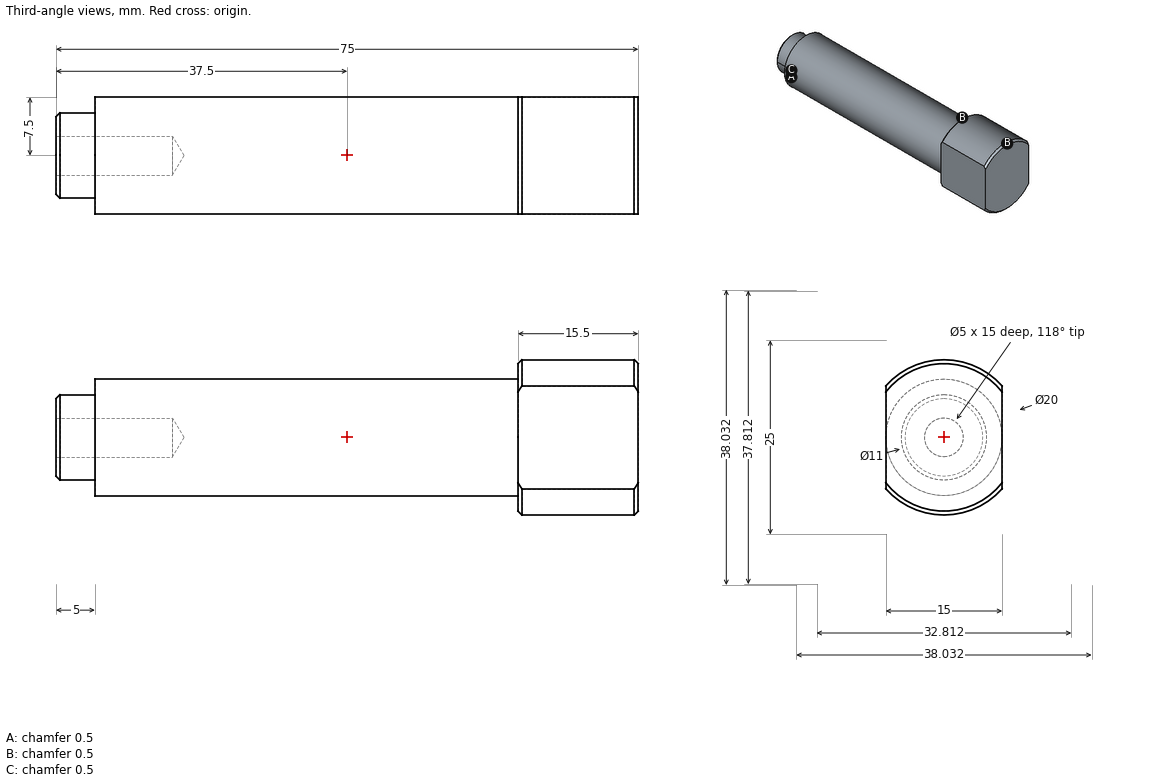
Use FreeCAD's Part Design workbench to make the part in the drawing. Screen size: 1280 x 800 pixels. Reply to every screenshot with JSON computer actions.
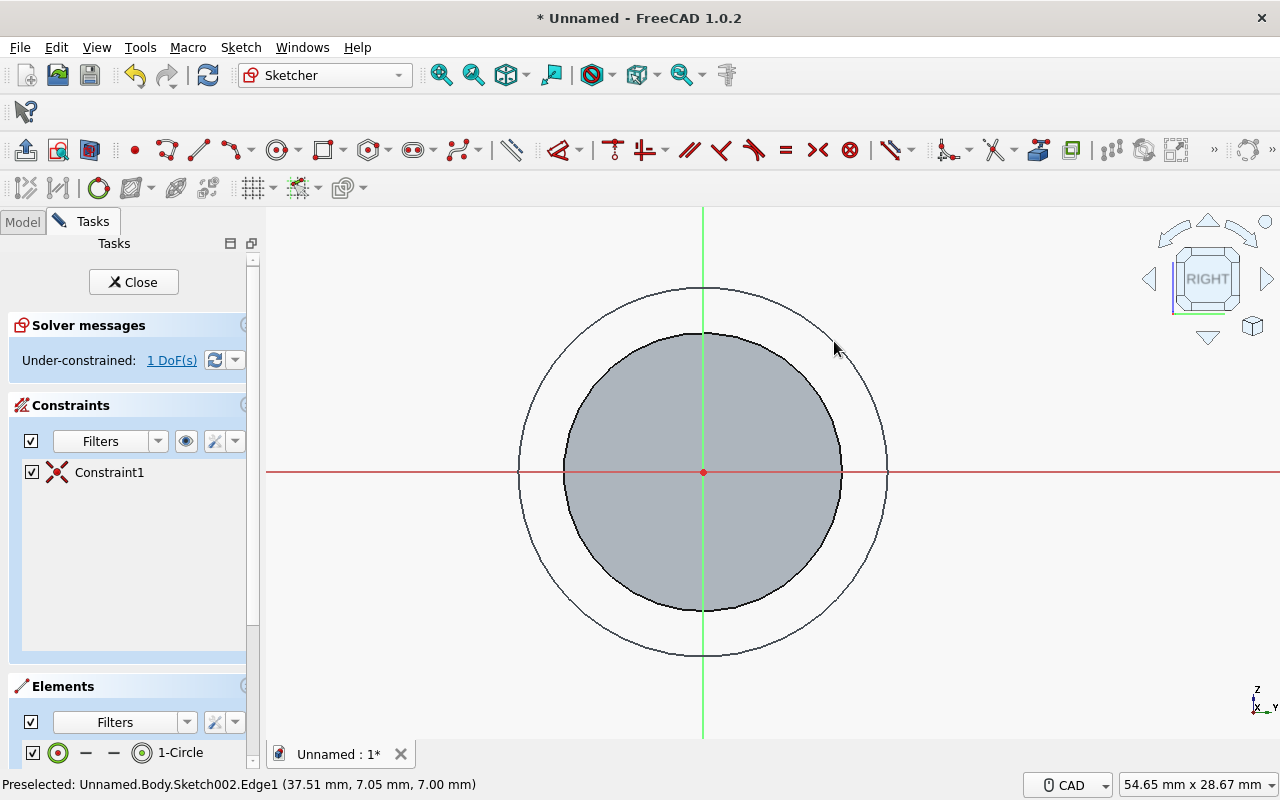
{"action": "left_click", "coordinate": [558, 150]}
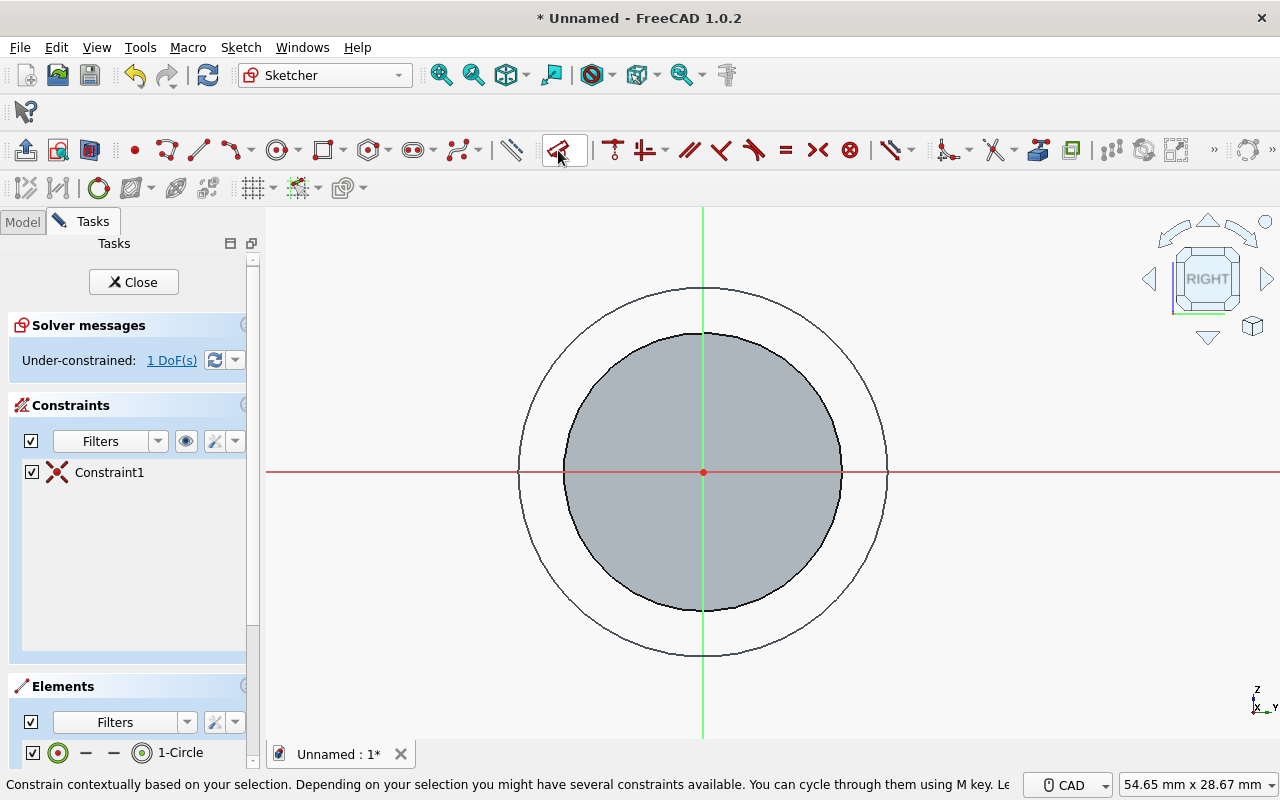
{"action": "left_click", "coordinate": [833, 341]}
{"action": "left_click", "coordinate": [856, 318]}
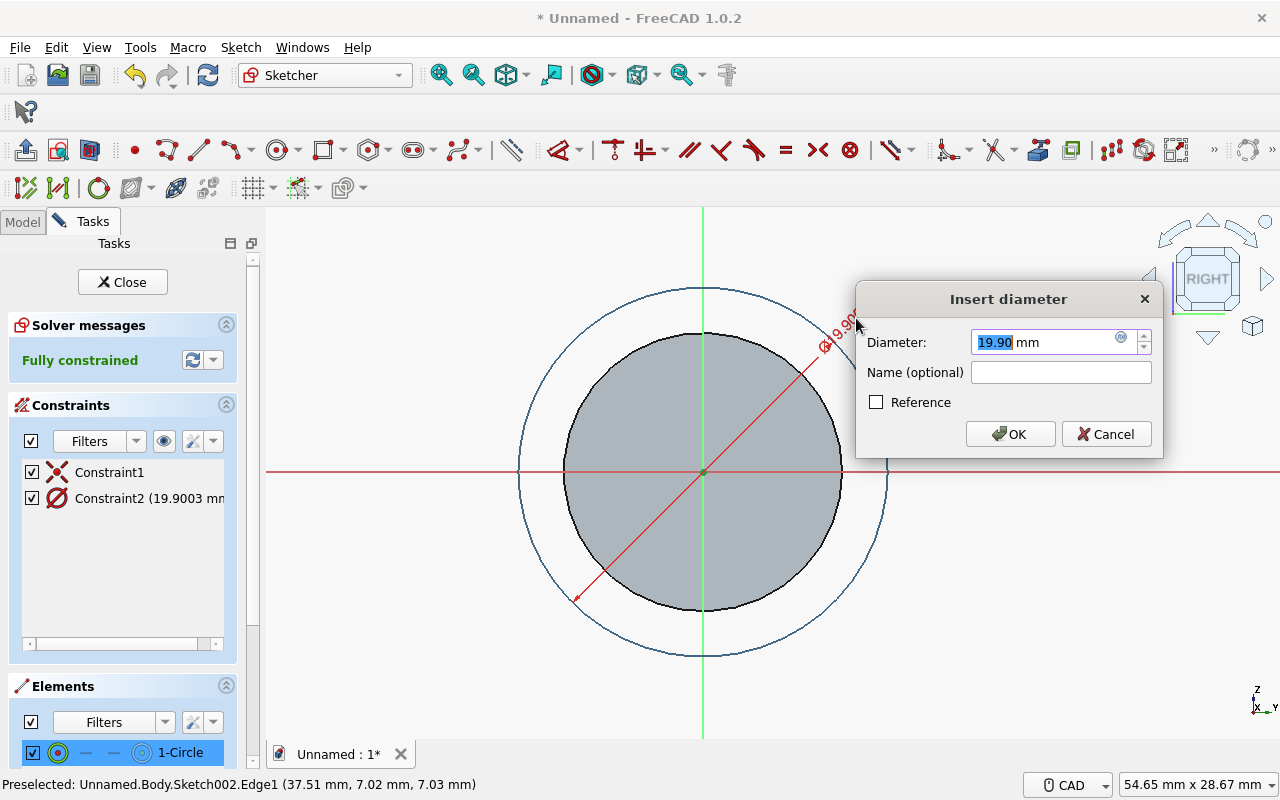
{"action": "type", "text": "20"}
{"action": "key", "text": "Return"}
{"action": "key", "text": "Escape"}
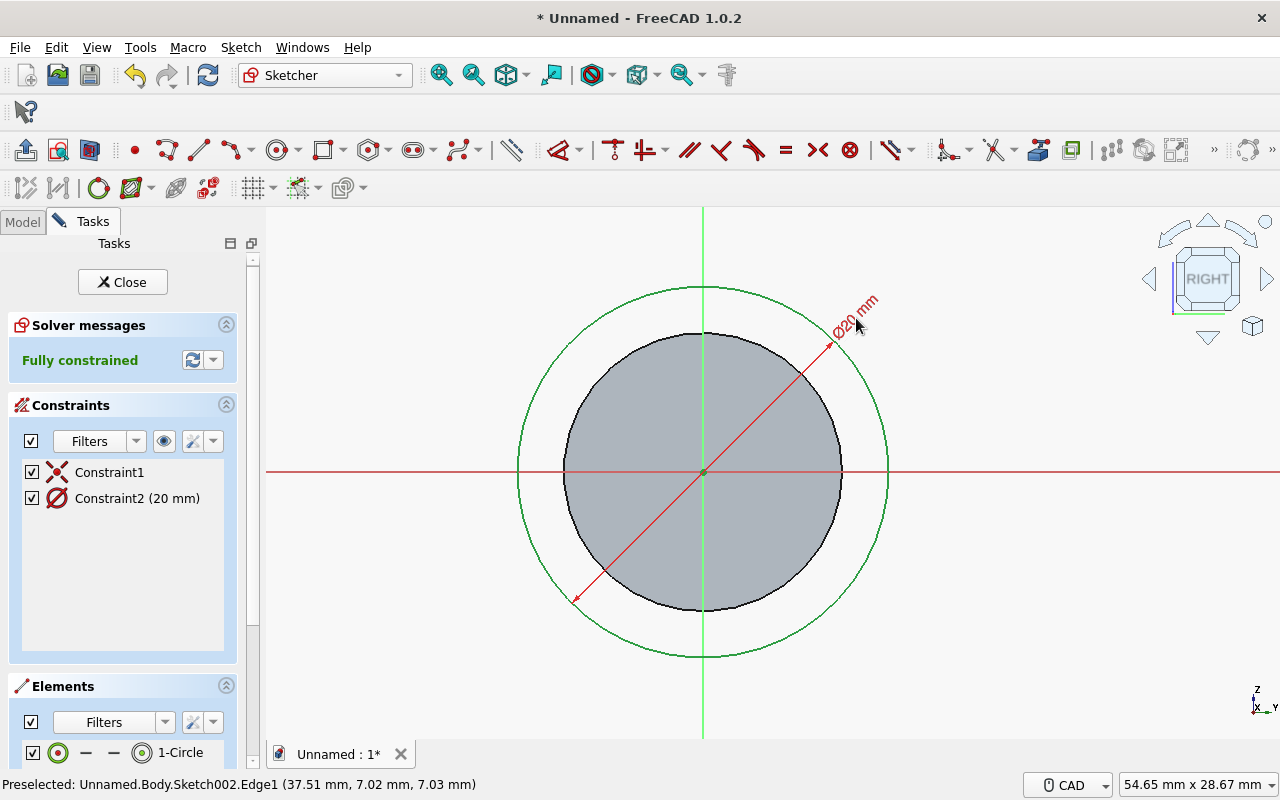
{"action": "left_click", "coordinate": [123, 282]}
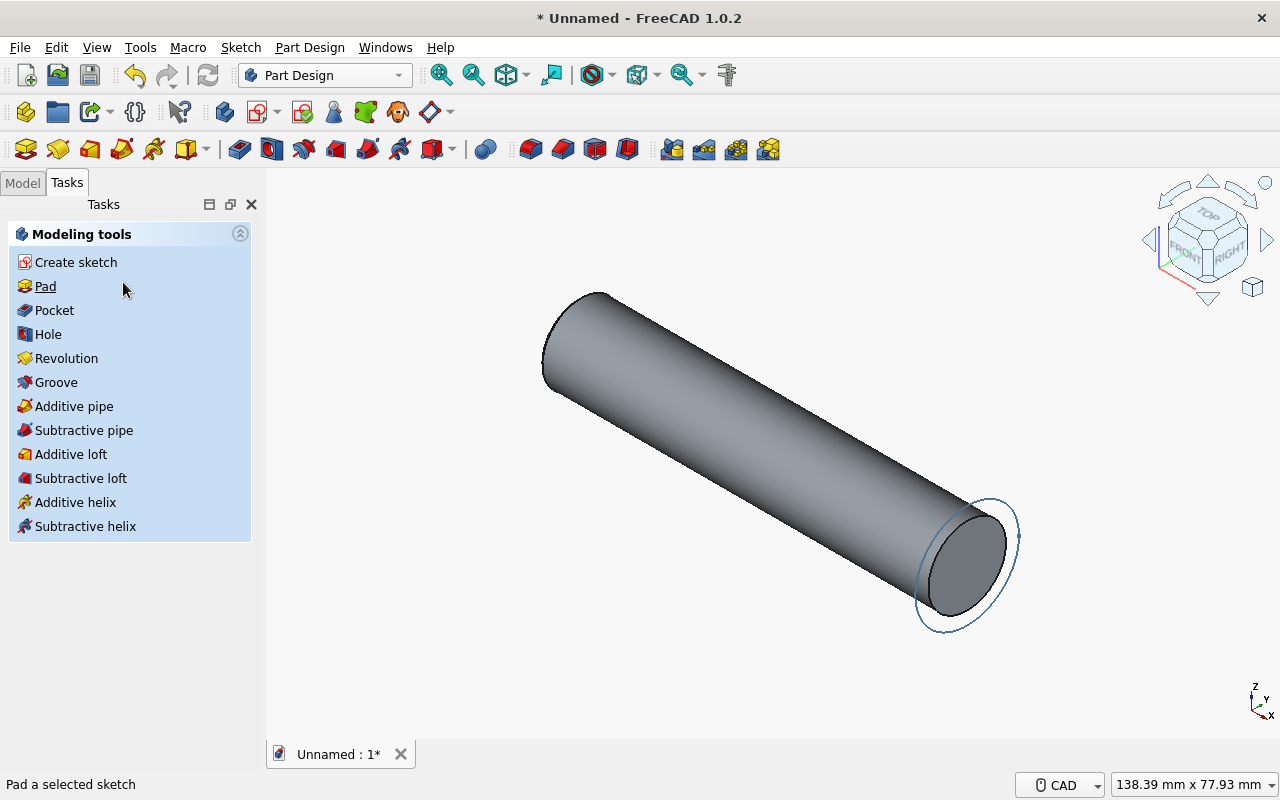
{"action": "left_click", "coordinate": [26, 150]}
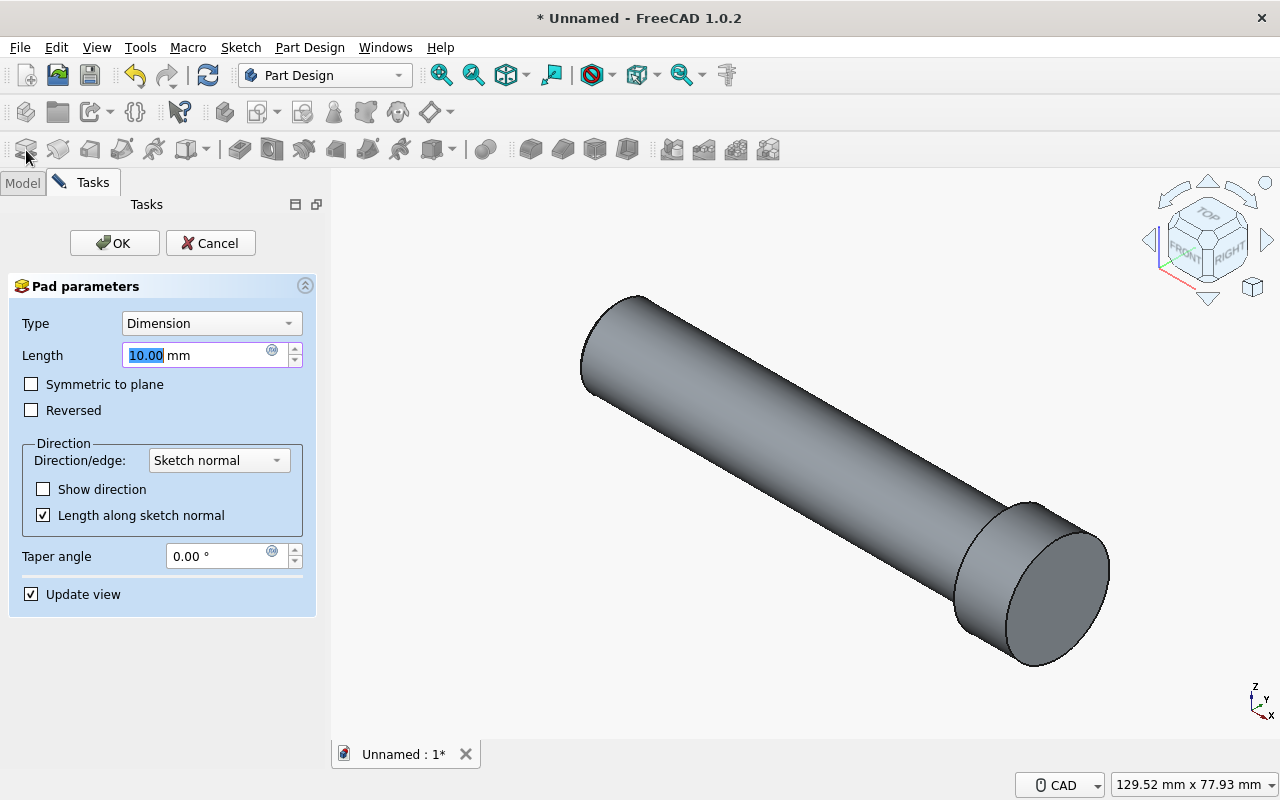
{"action": "type", "text": "15.5"}
{"action": "key", "text": "Tab"}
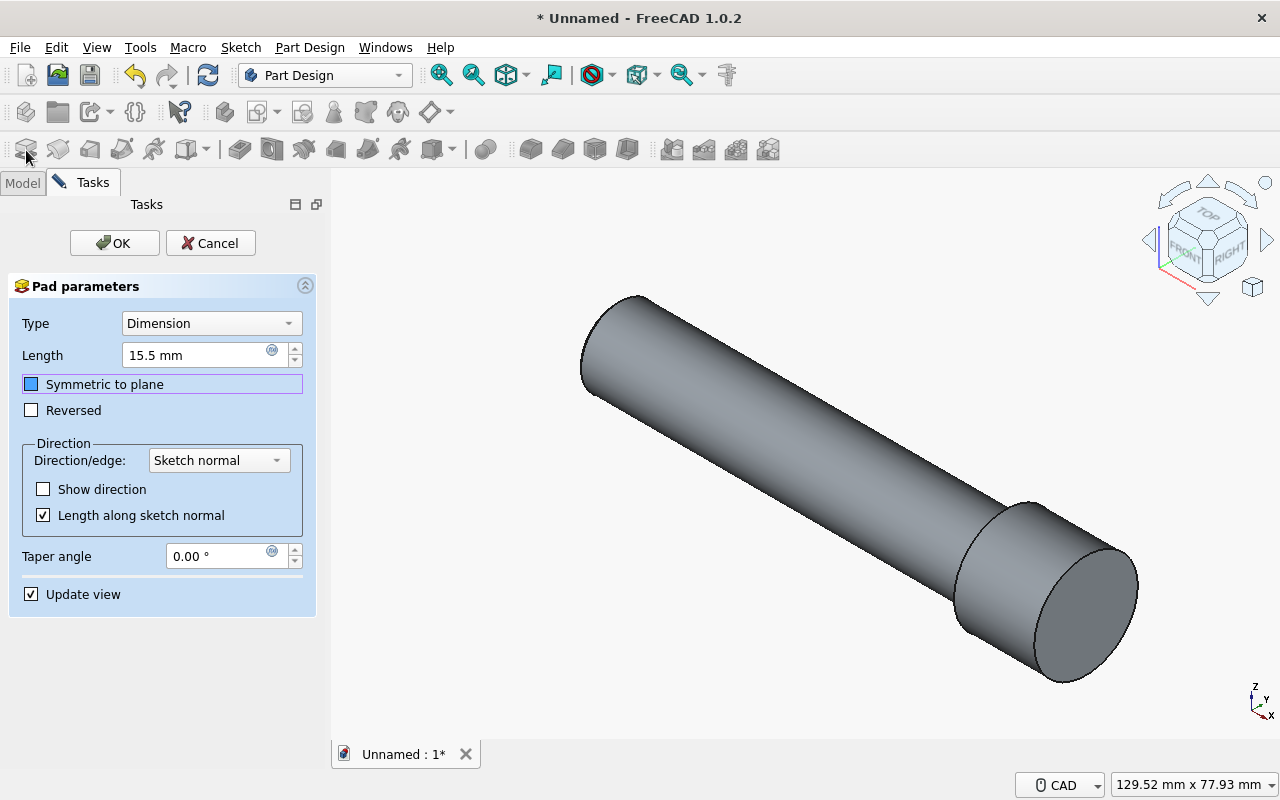
{"action": "left_click", "coordinate": [30, 410]}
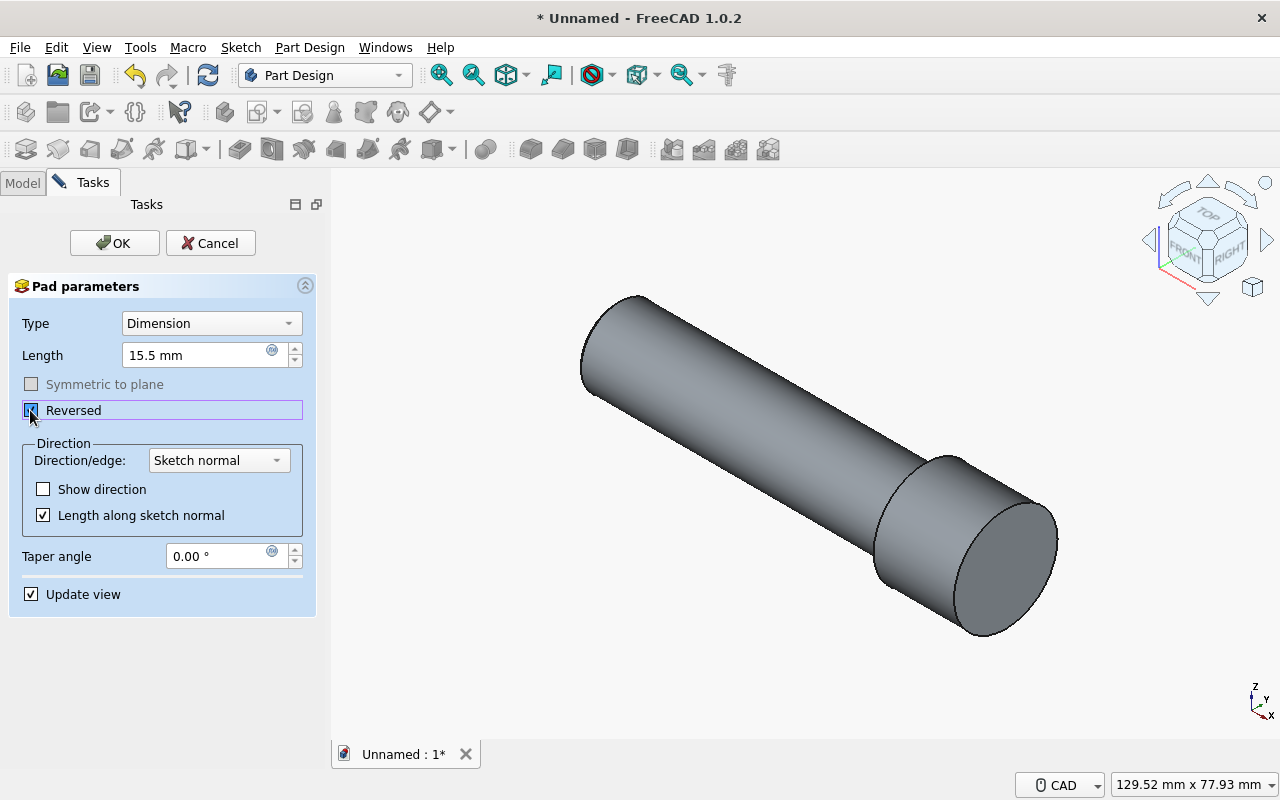
{"action": "left_click", "coordinate": [115, 243]}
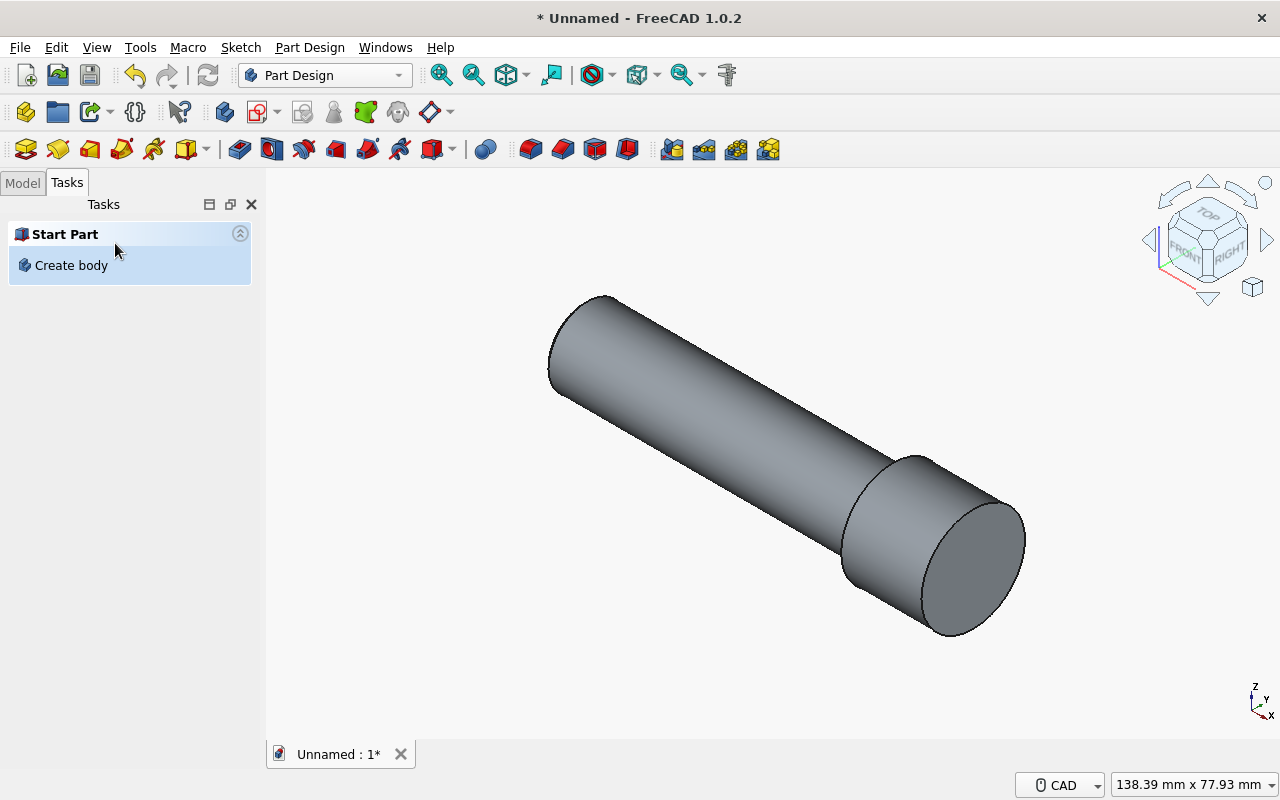
{"action": "left_click", "coordinate": [877, 474]}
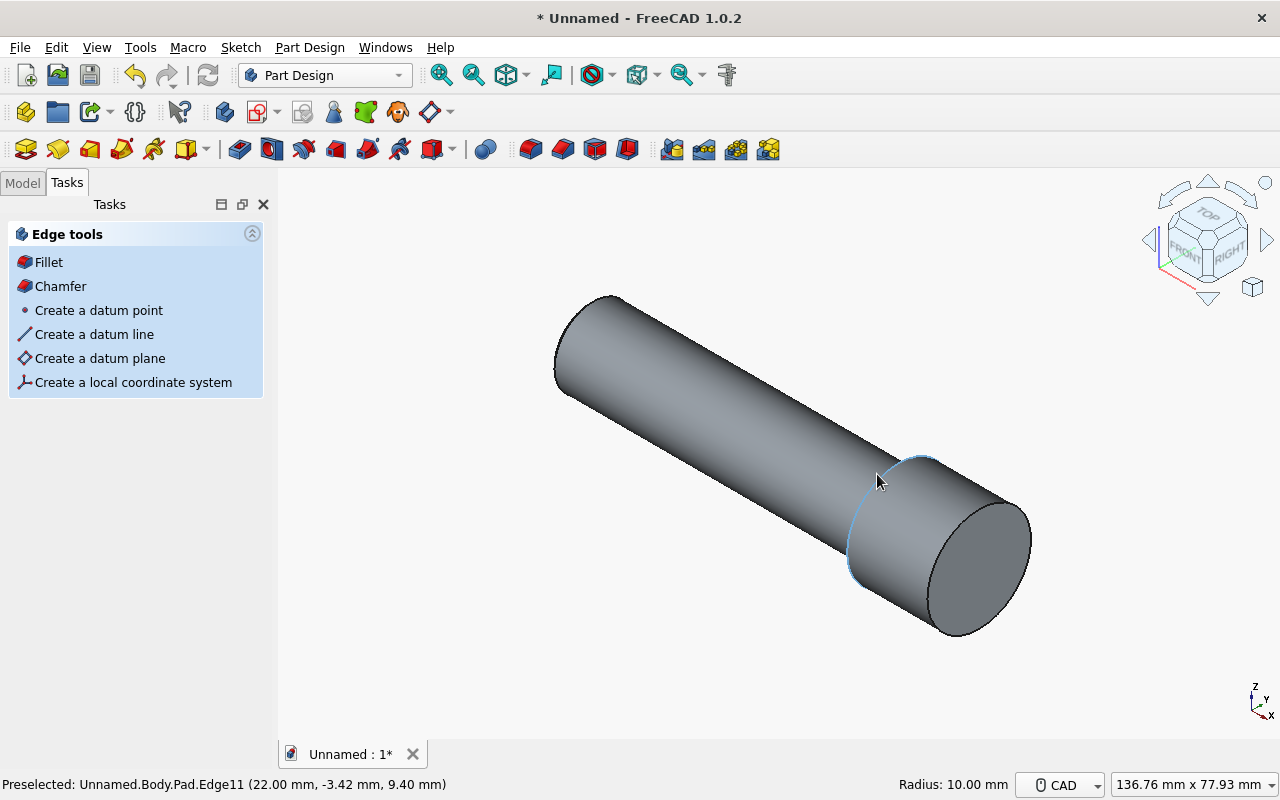
{"action": "left_click", "coordinate": [927, 598], "text": "ctrl"}